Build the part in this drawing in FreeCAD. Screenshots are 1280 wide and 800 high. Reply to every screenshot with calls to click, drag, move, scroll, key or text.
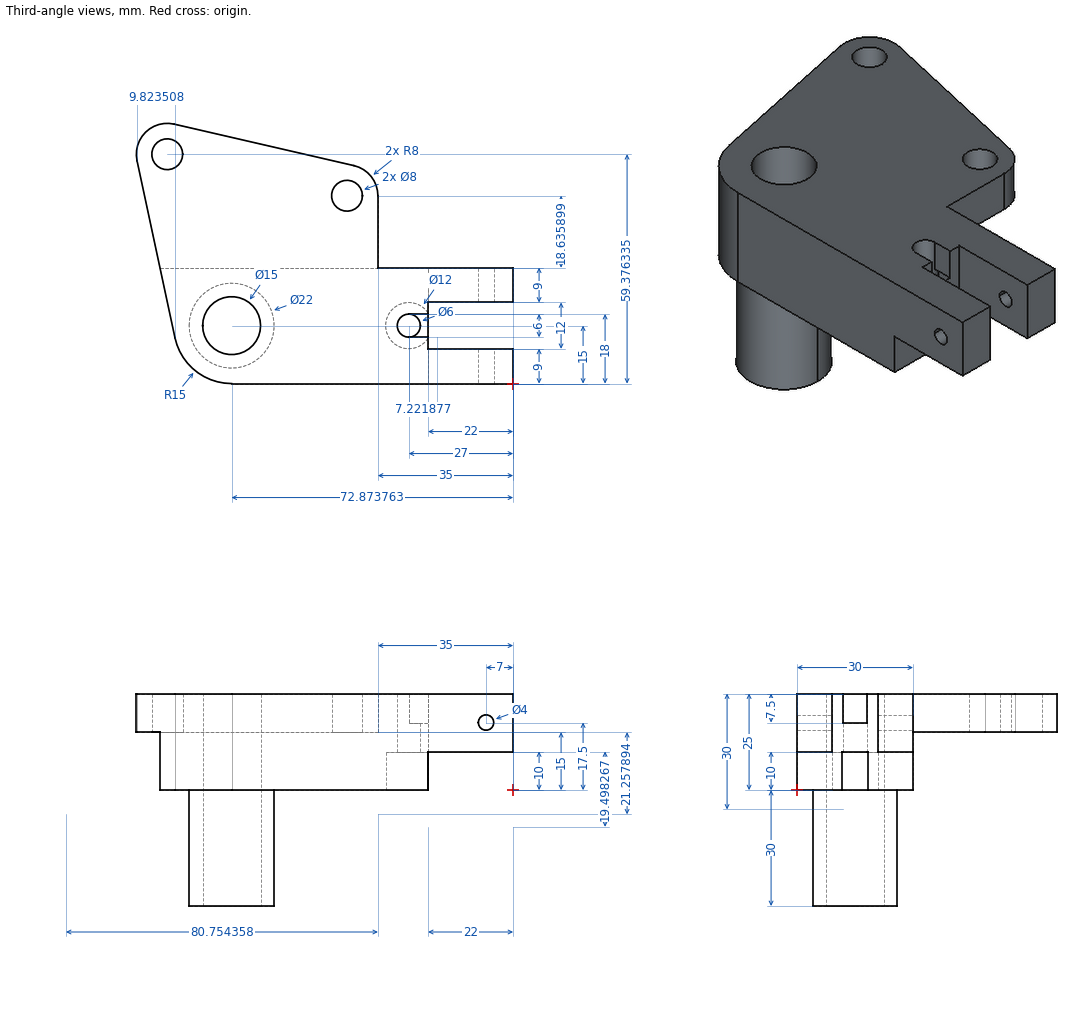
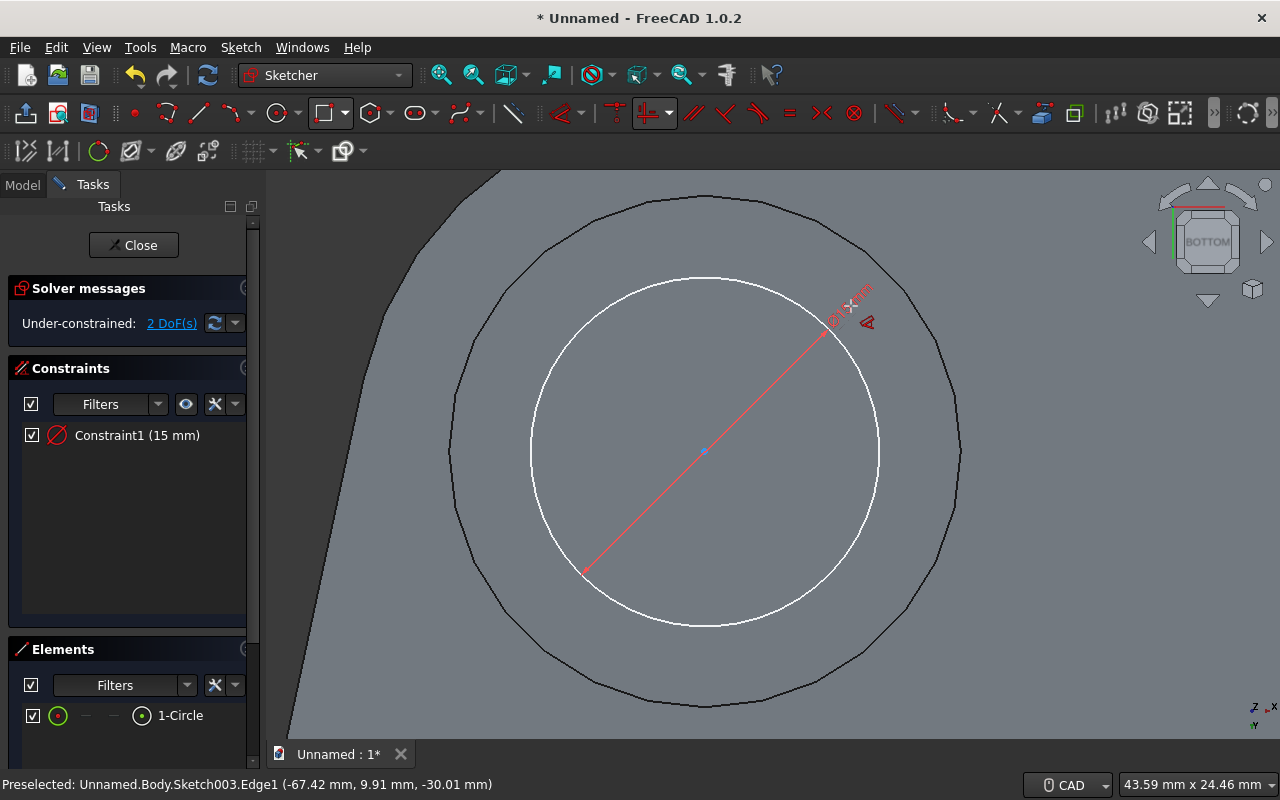
click(705, 452)
click(671, 325)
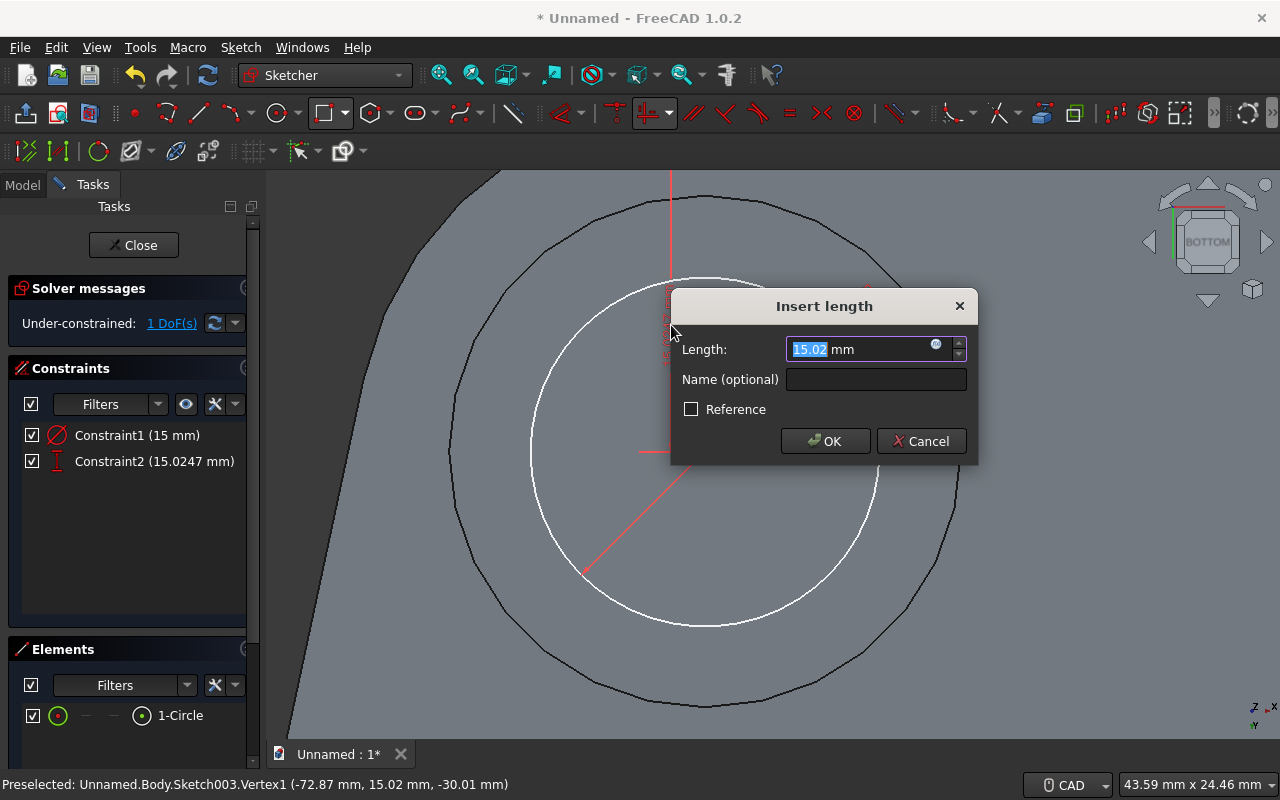
text(15)
key(Return)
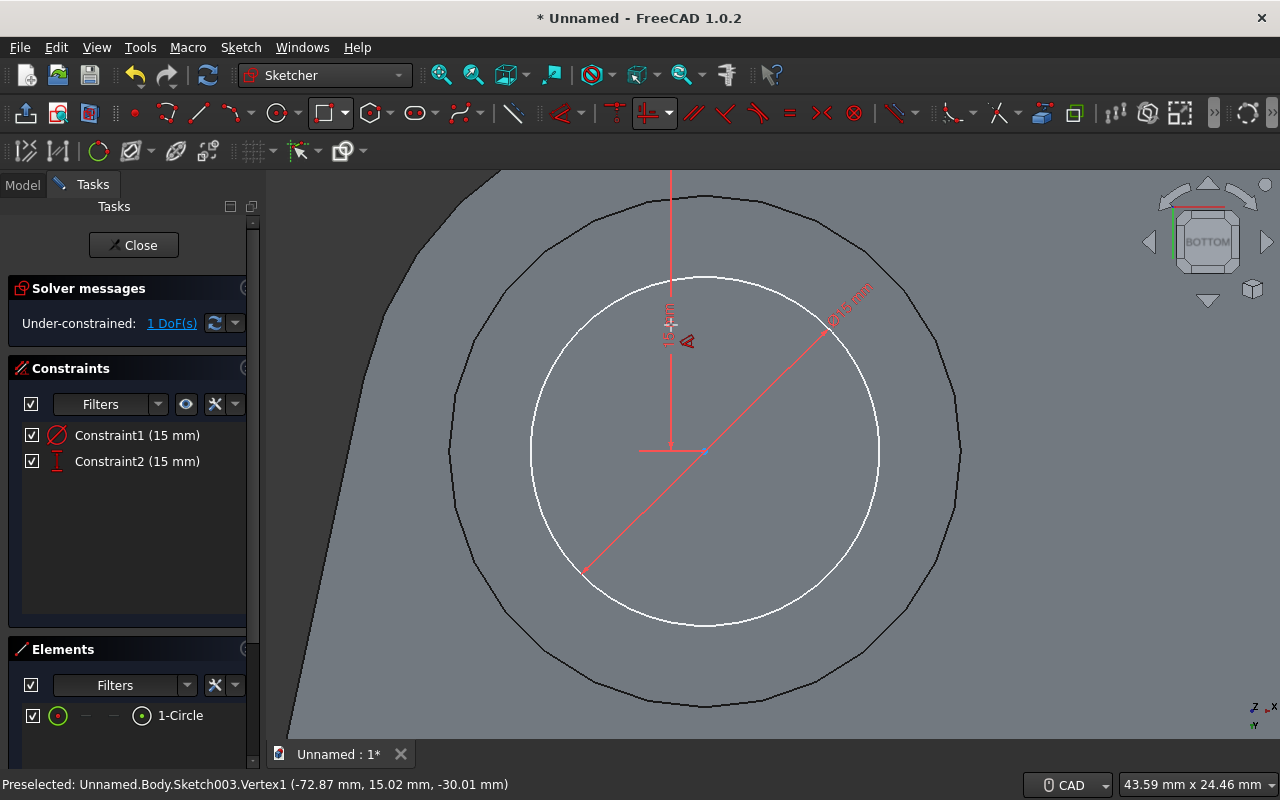
click(705, 451)
click(910, 485)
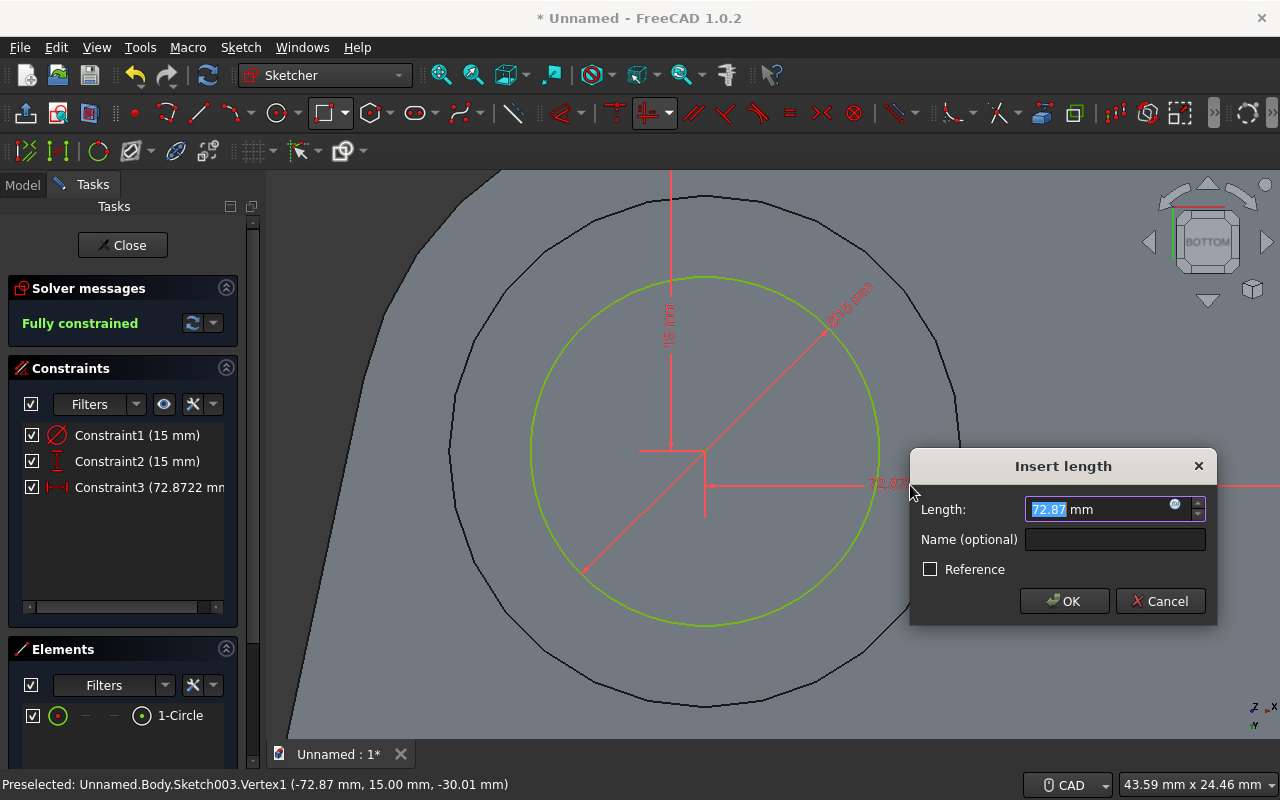
text(72.873763)
key(Return)
key(Escape)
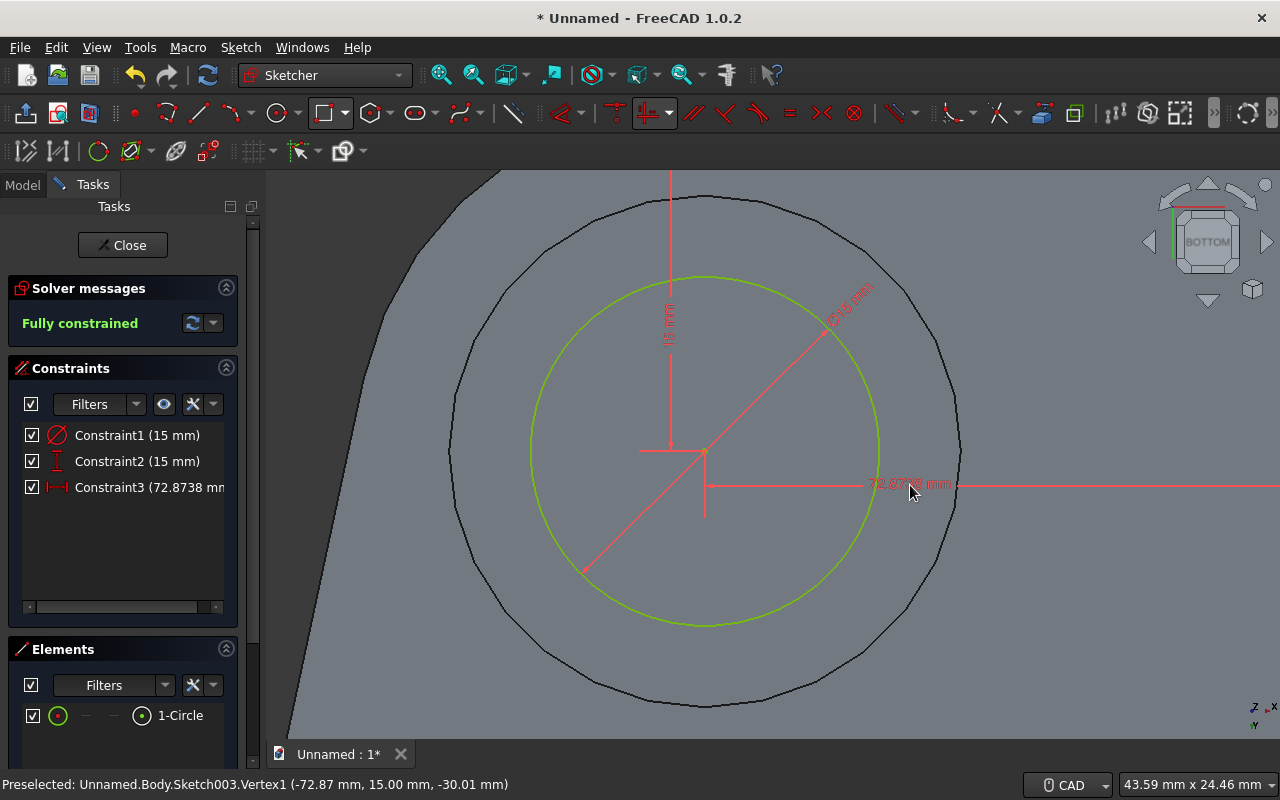
click(123, 245)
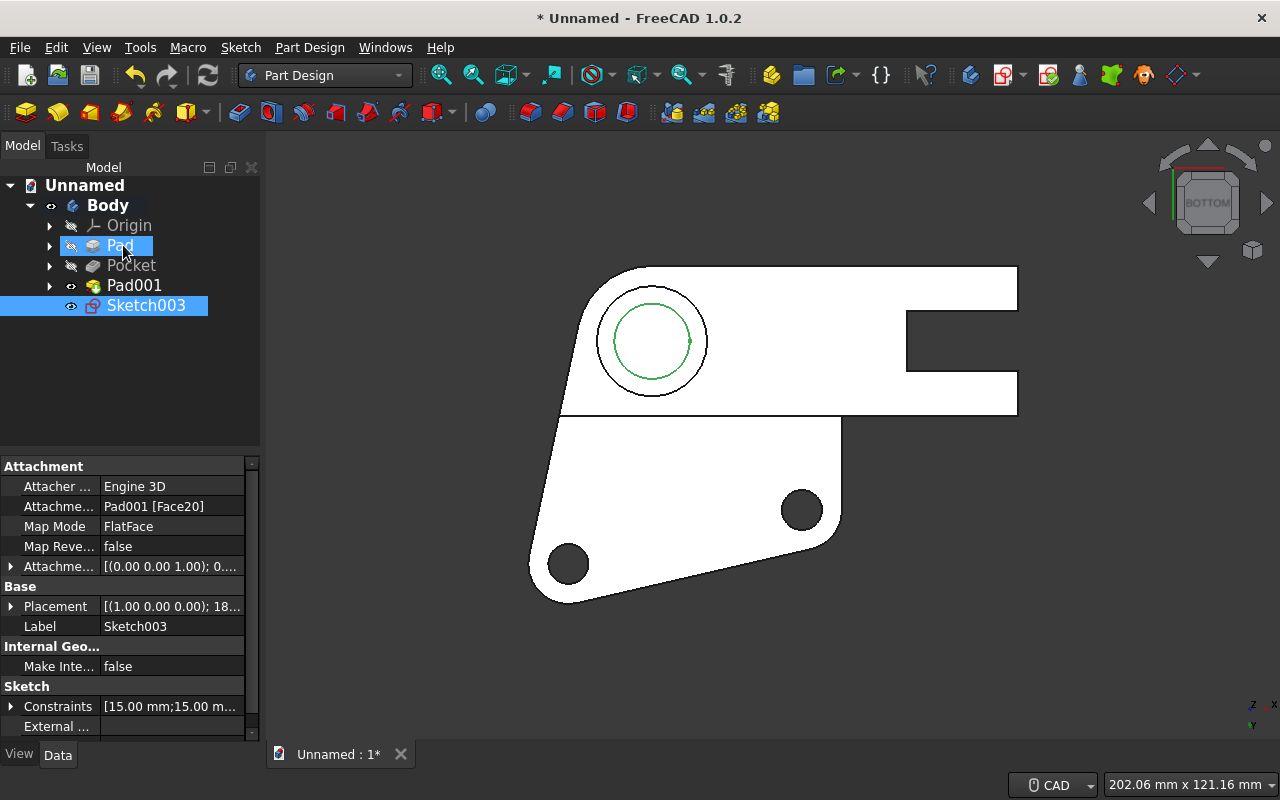
click(240, 112)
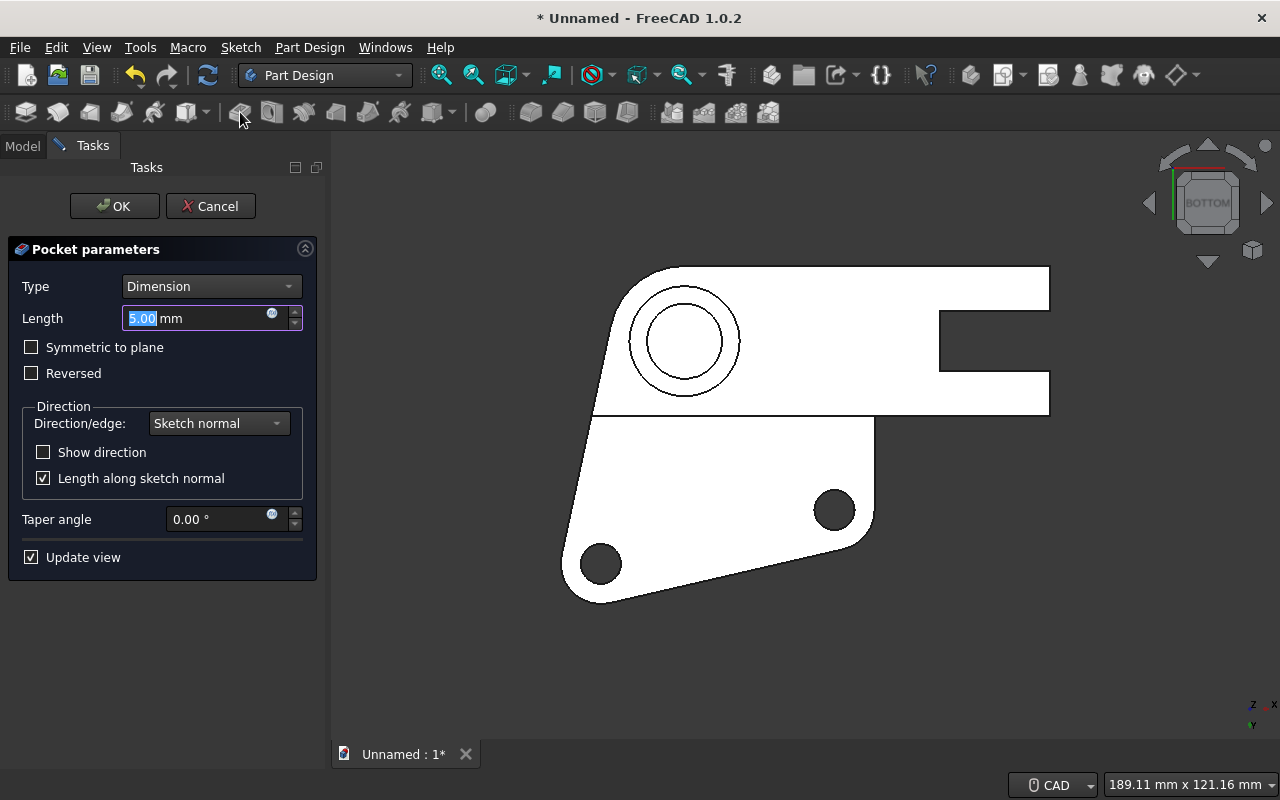
click(212, 286)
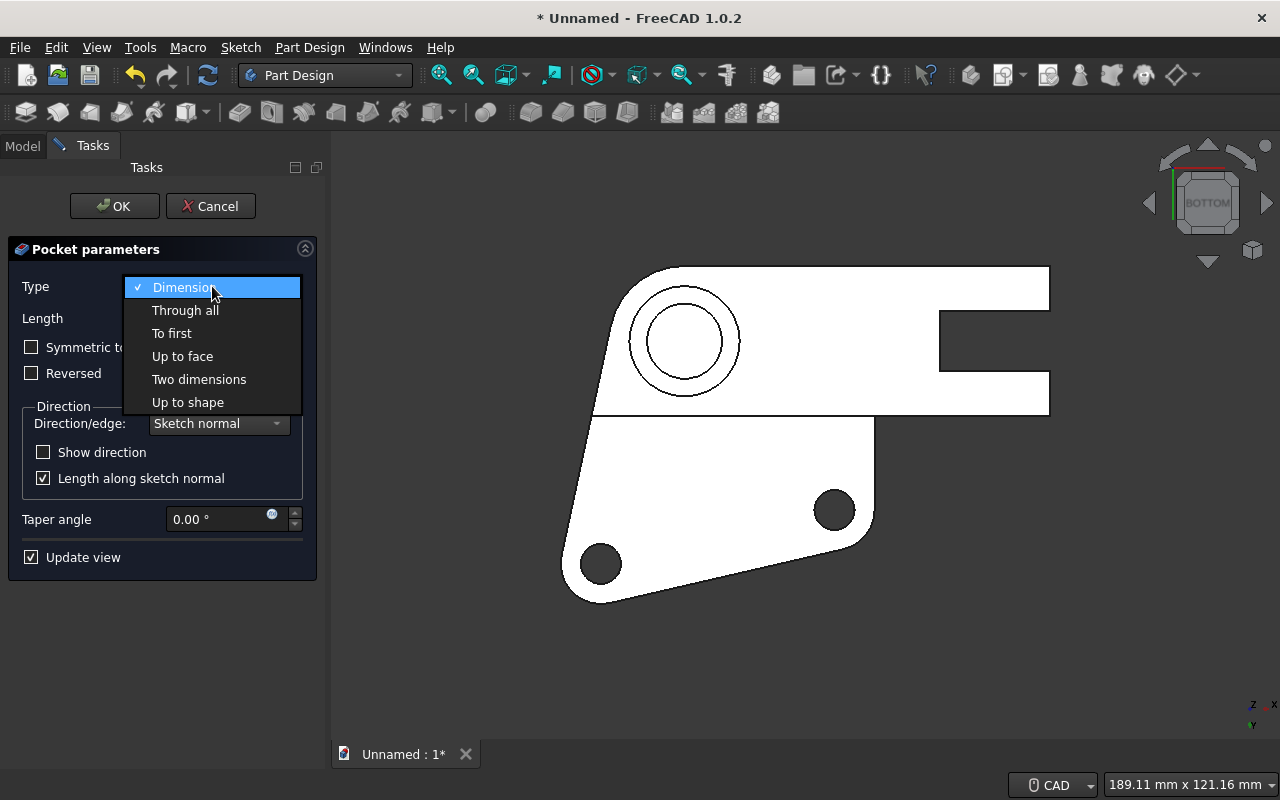
click(212, 310)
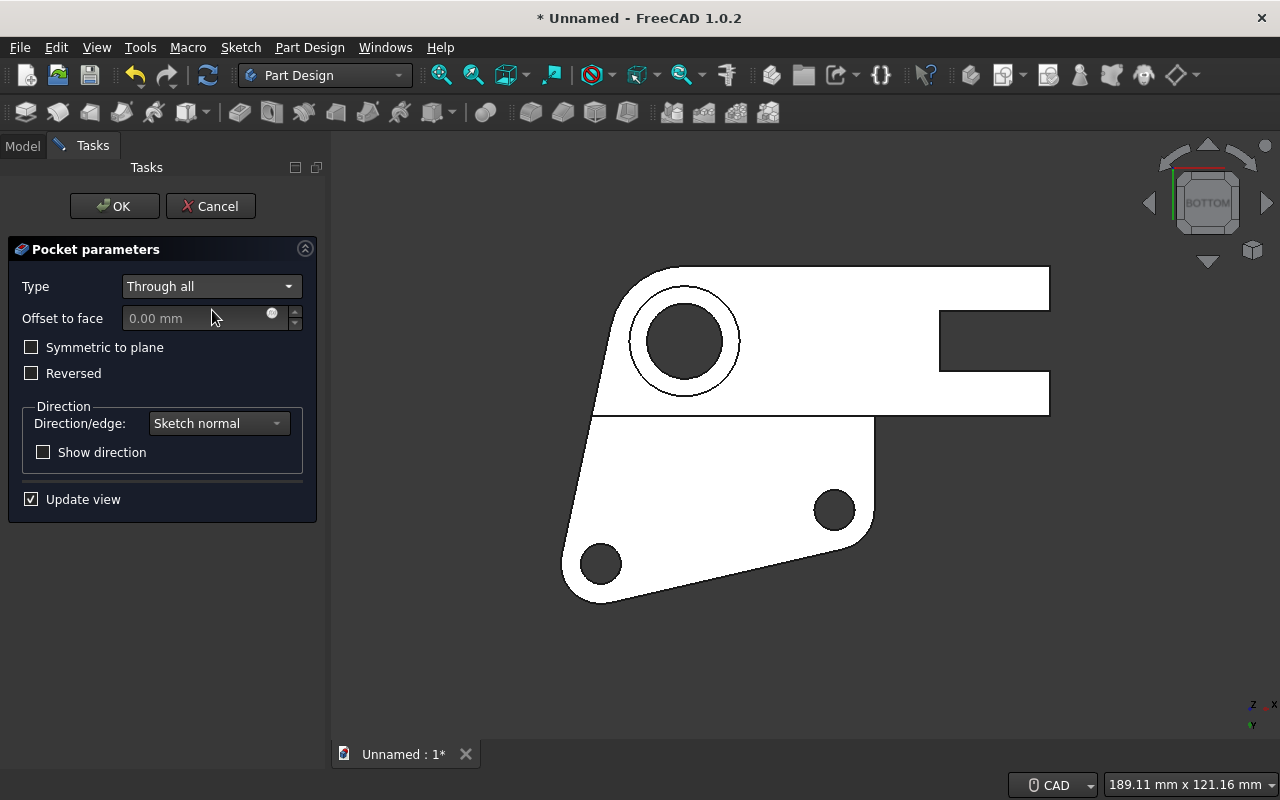
click(115, 206)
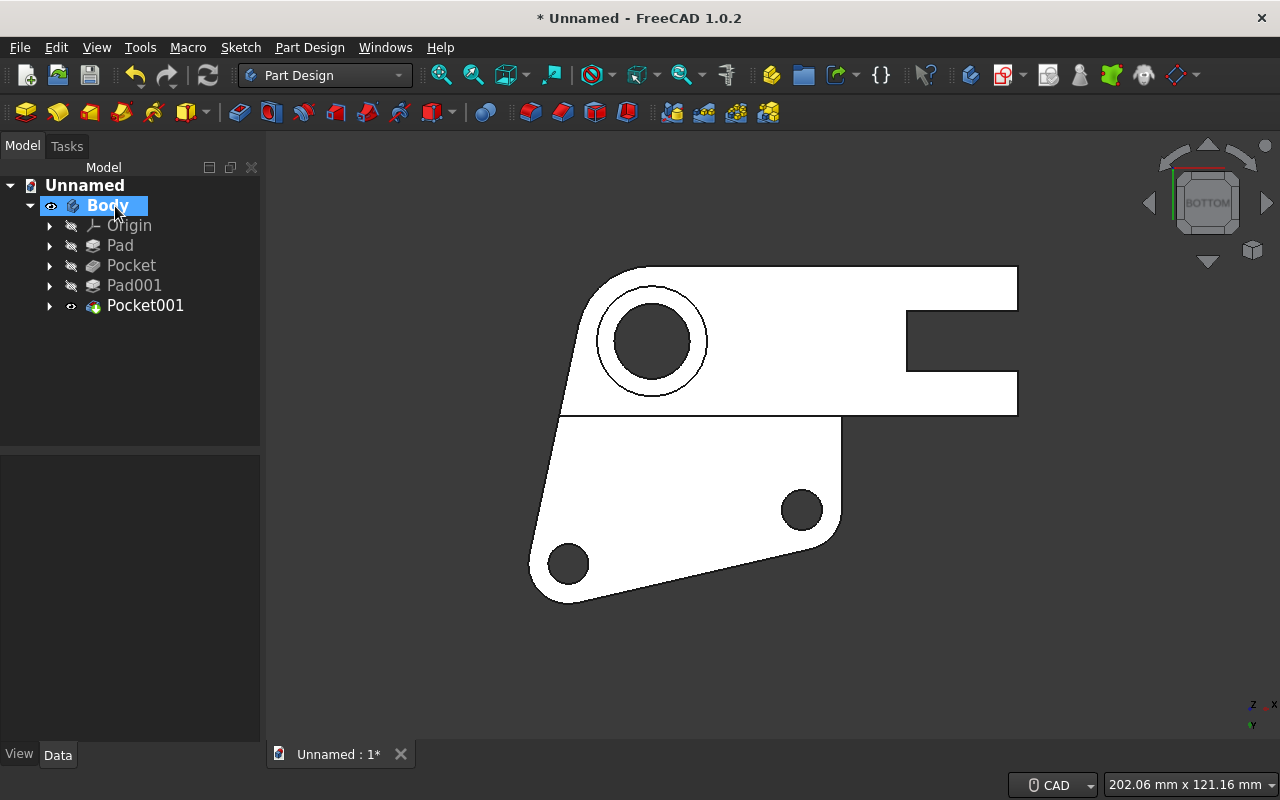
key(4)